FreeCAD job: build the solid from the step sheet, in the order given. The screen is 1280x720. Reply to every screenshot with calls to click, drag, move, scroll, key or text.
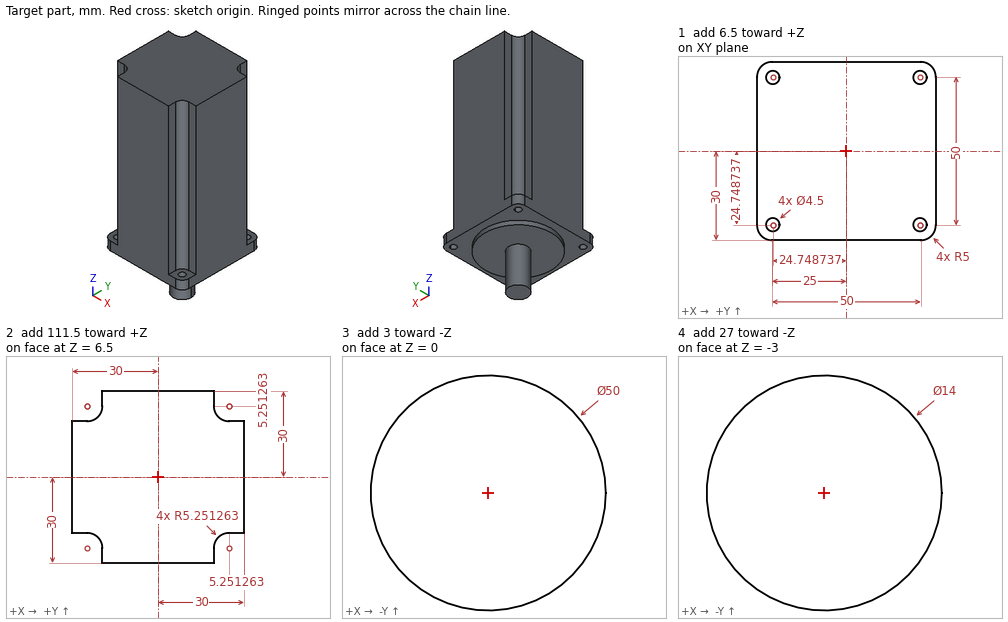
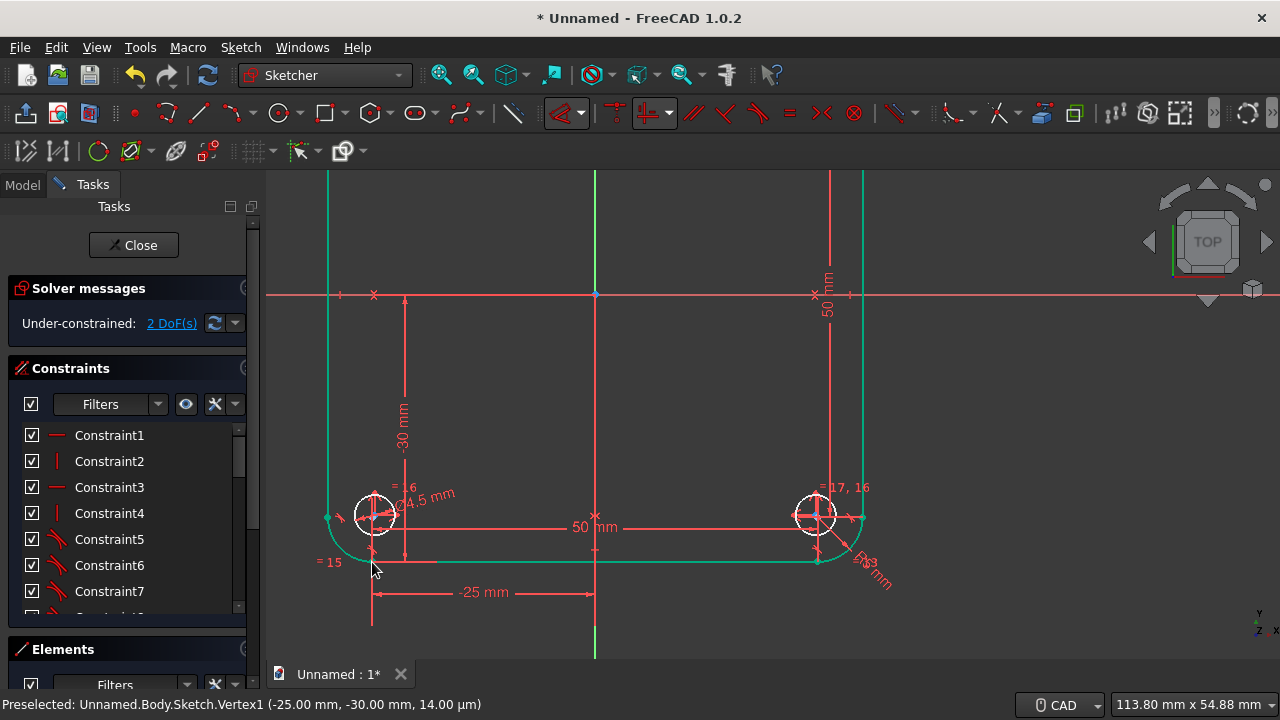
scroll(375, 515, up, 7)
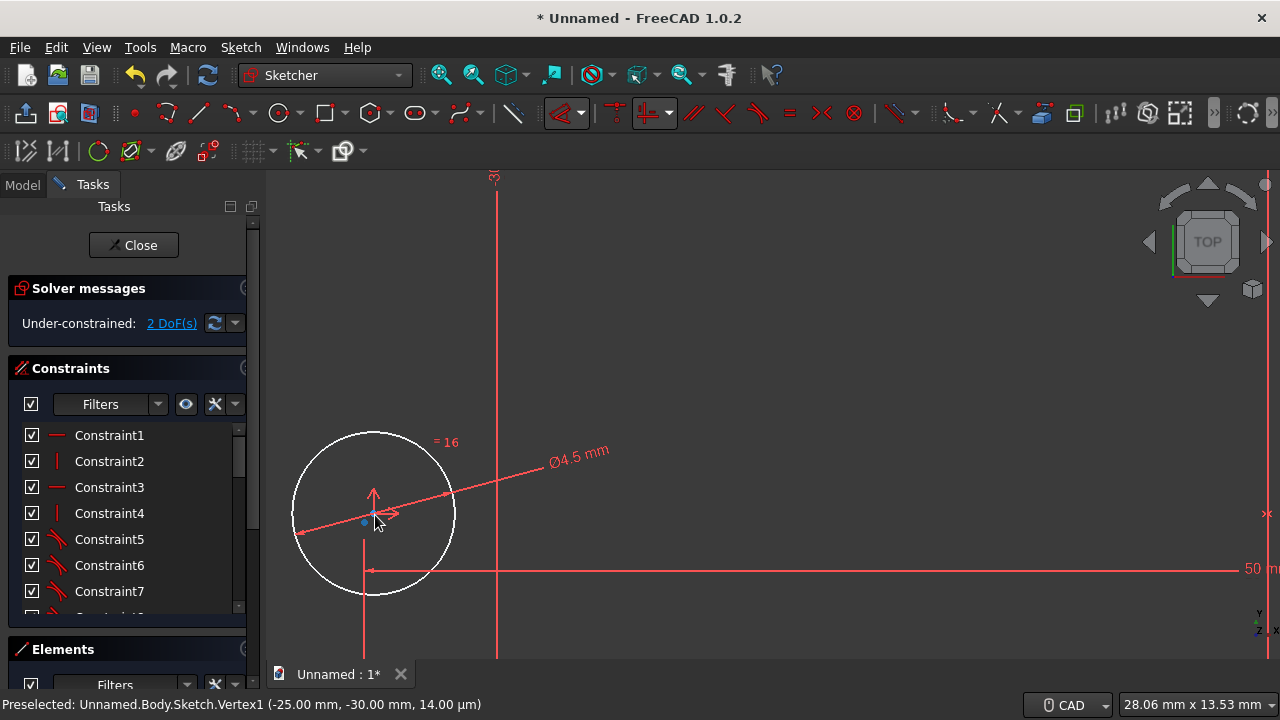
click(374, 514)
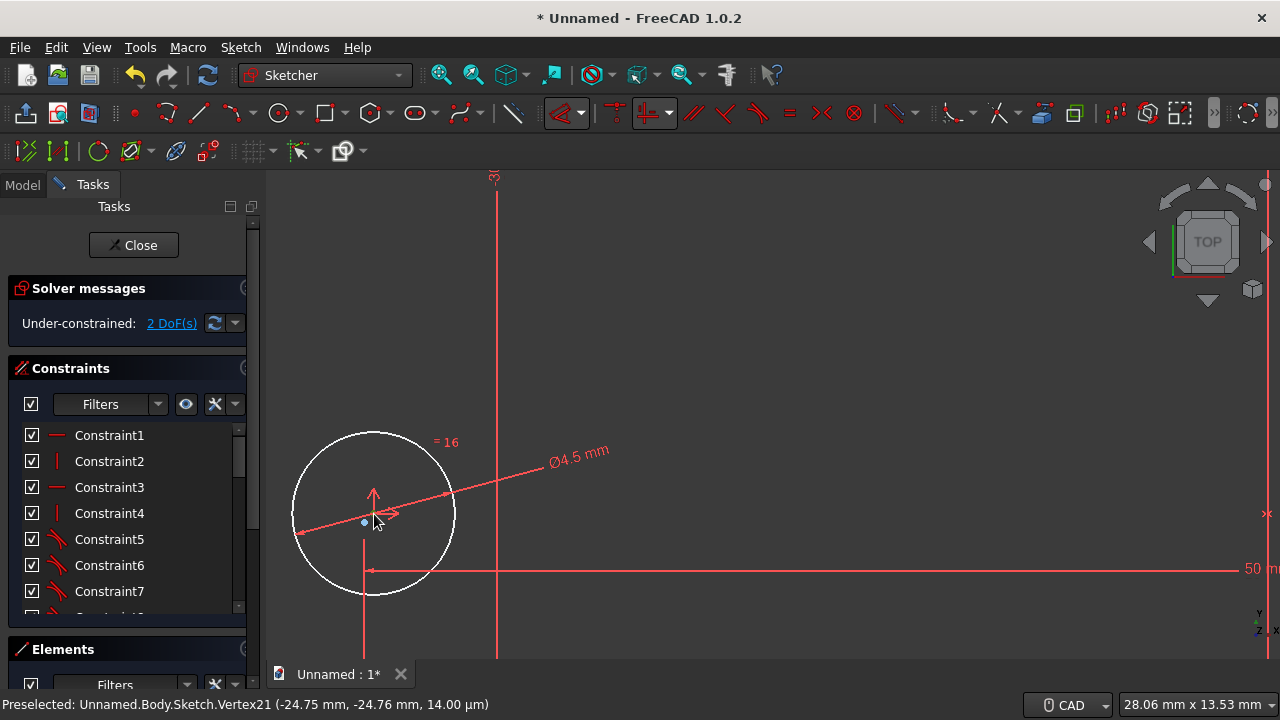
key(l)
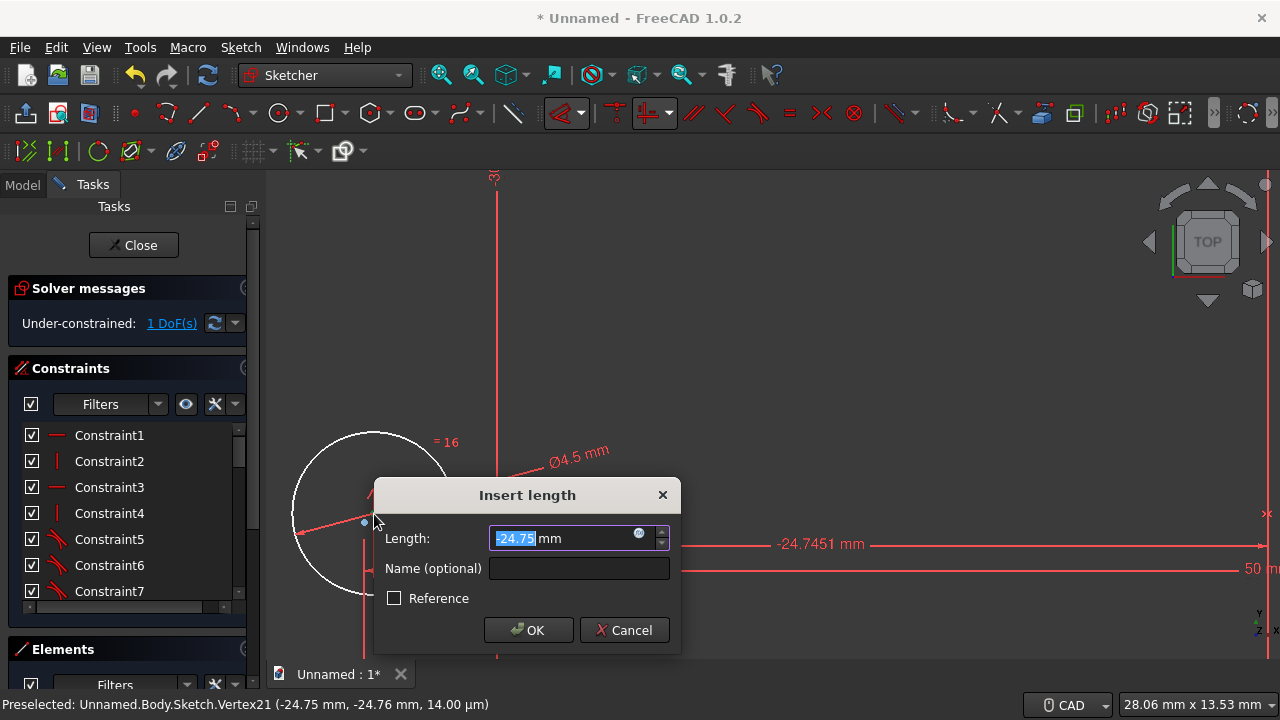
text(-24.748737)
key(Return)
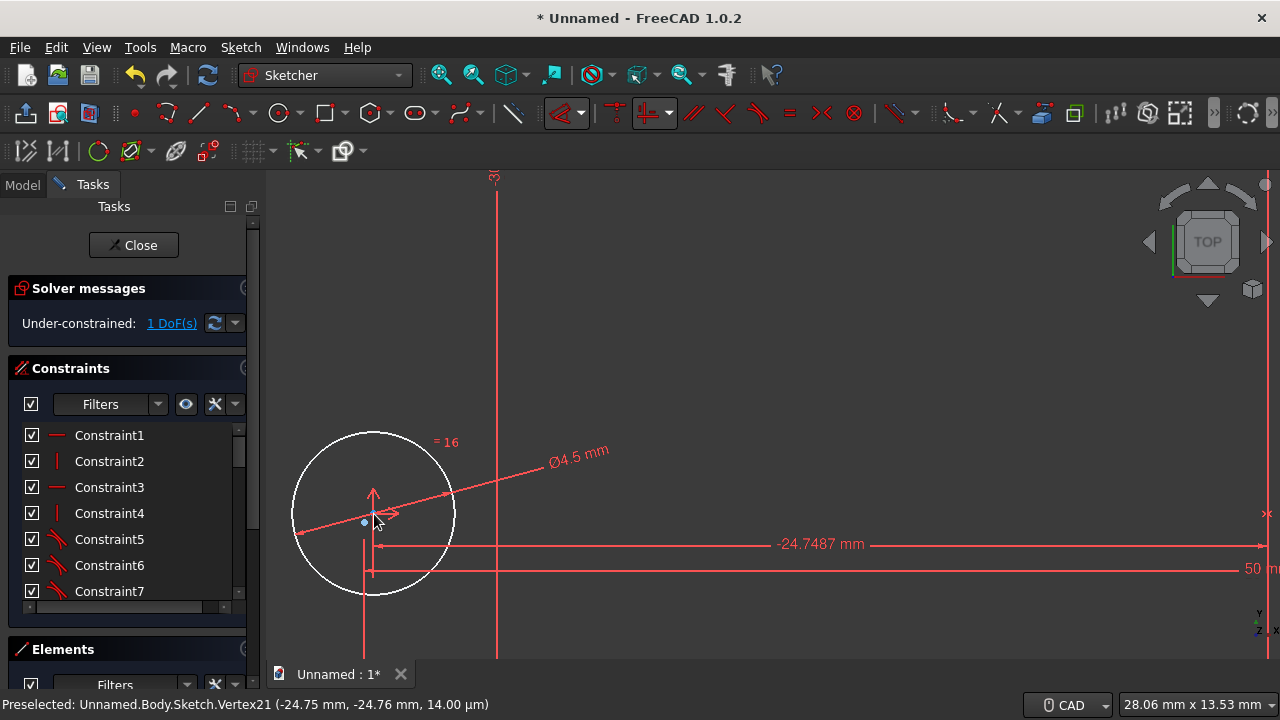
click(373, 514)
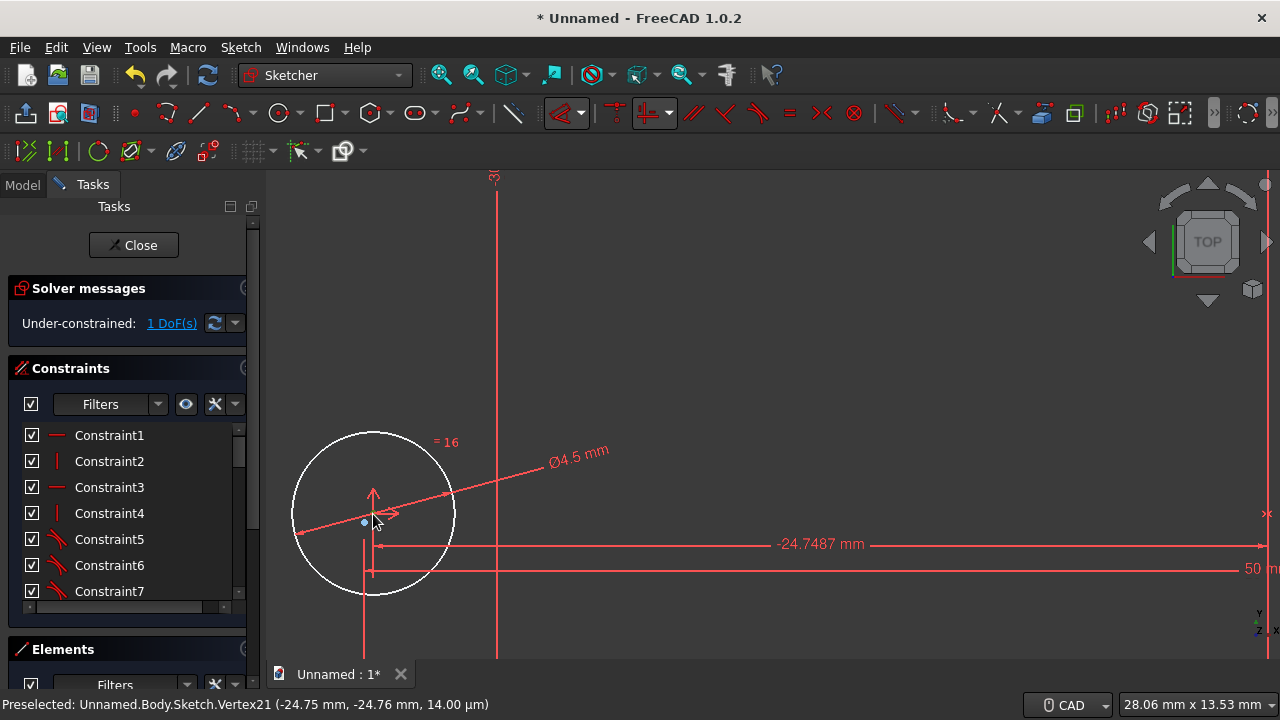
click(584, 114)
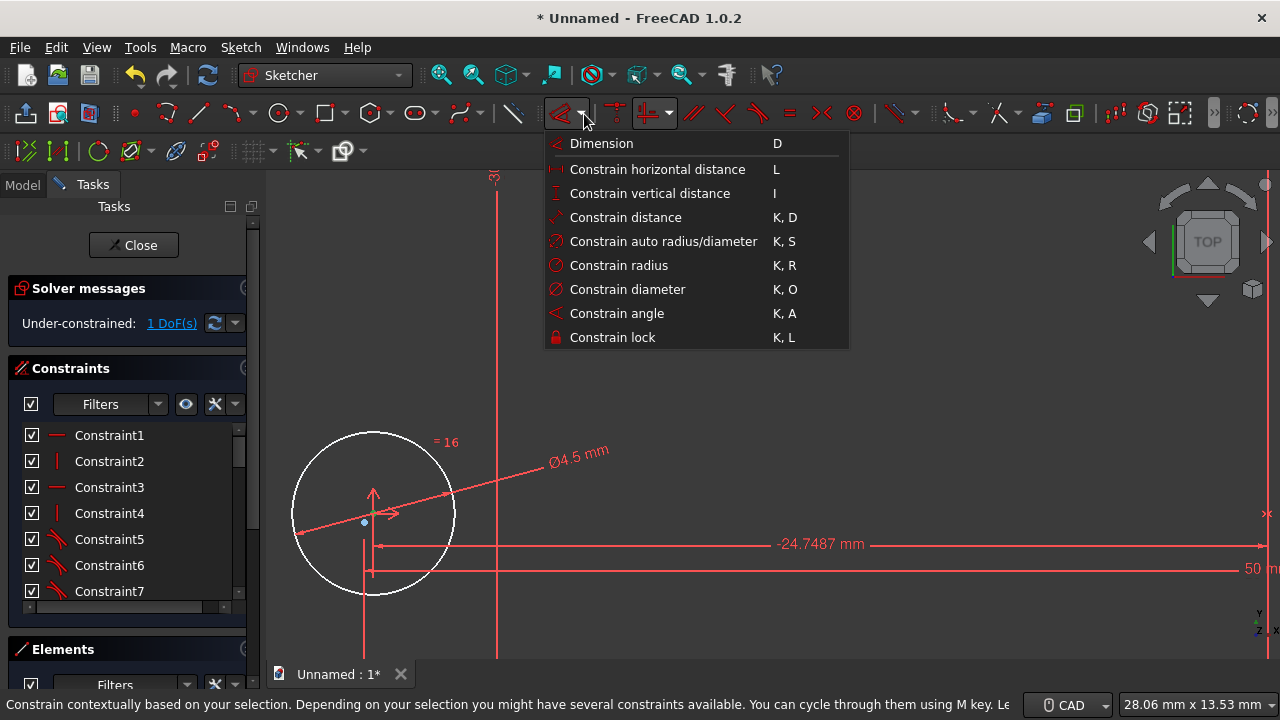
click(697, 193)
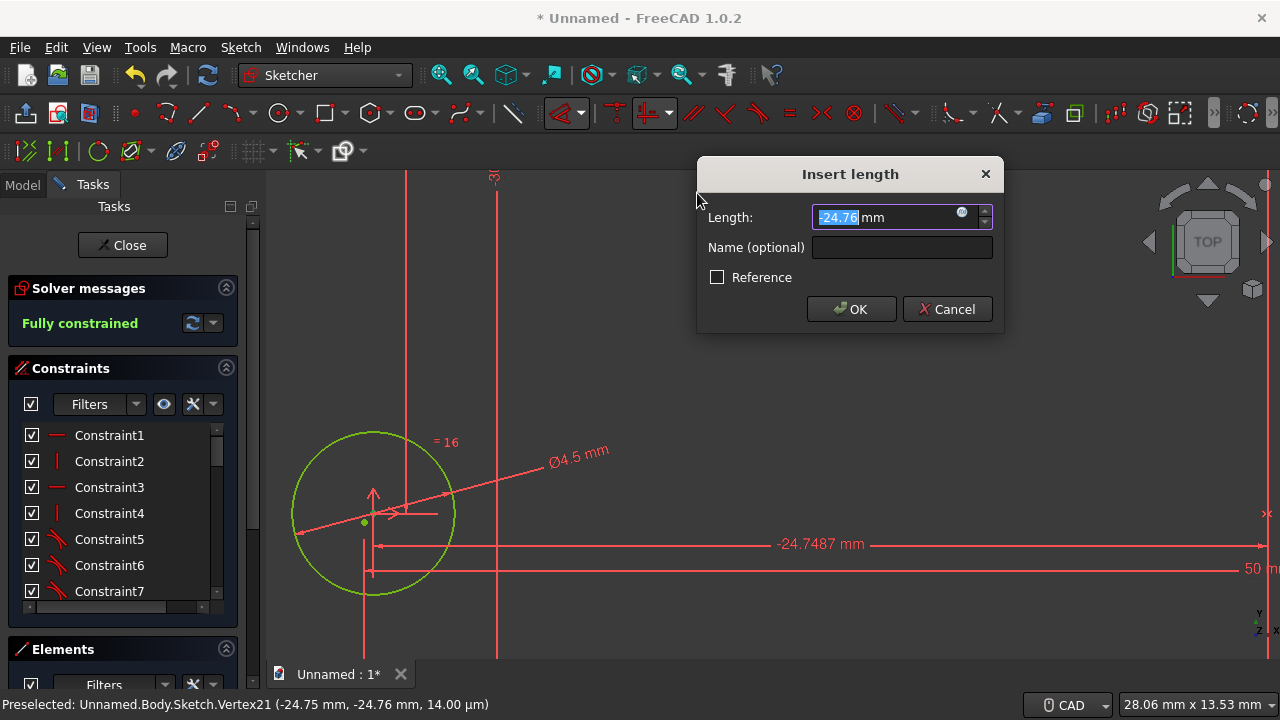
text(-24.748737)
key(Return)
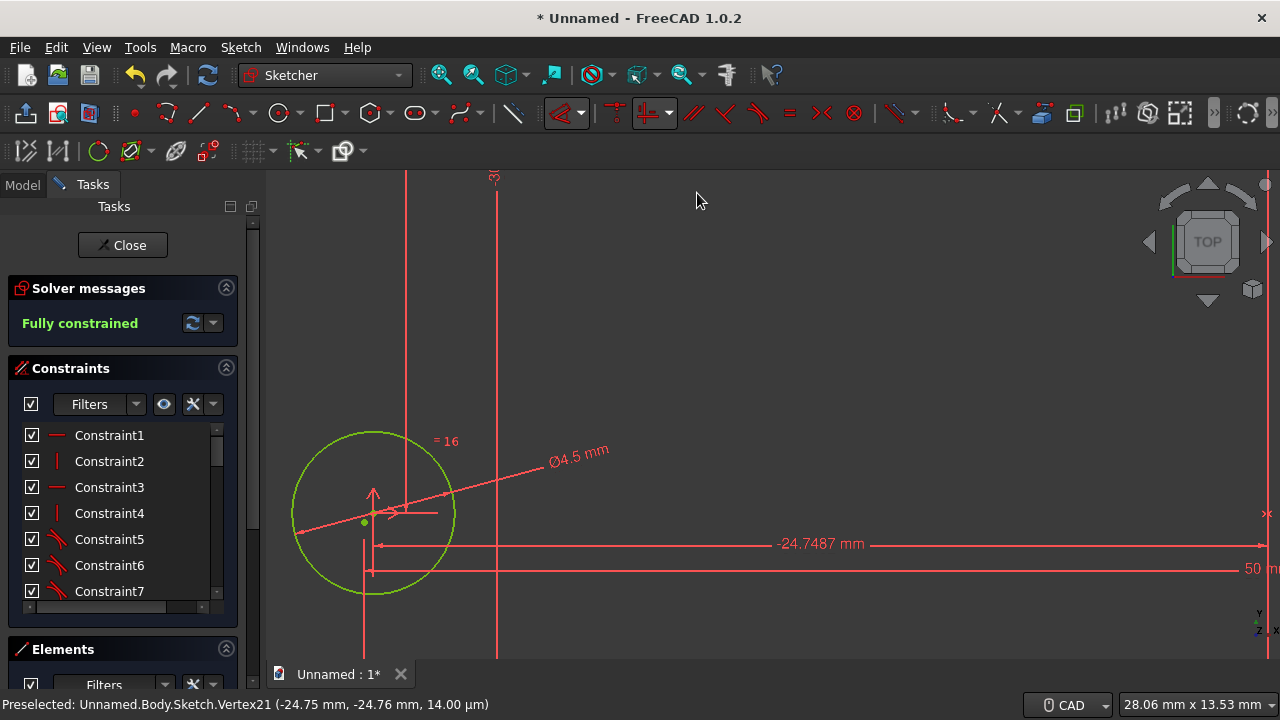
click(123, 245)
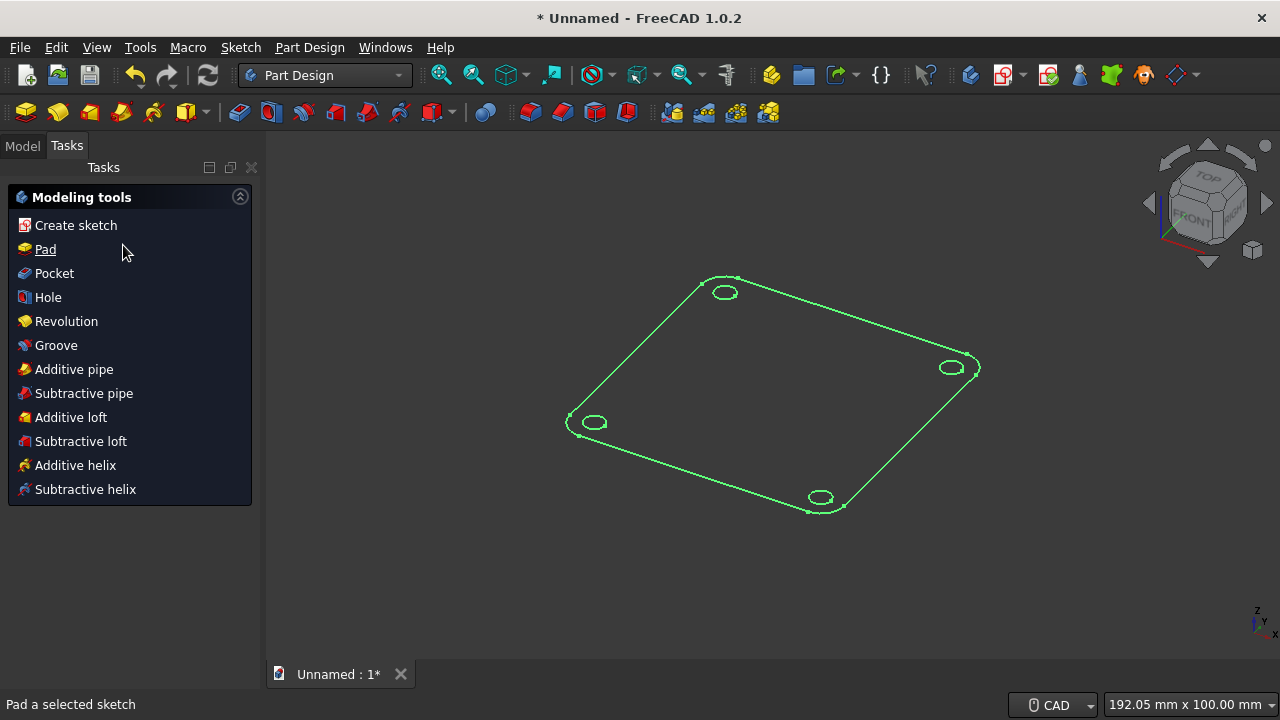
click(26, 112)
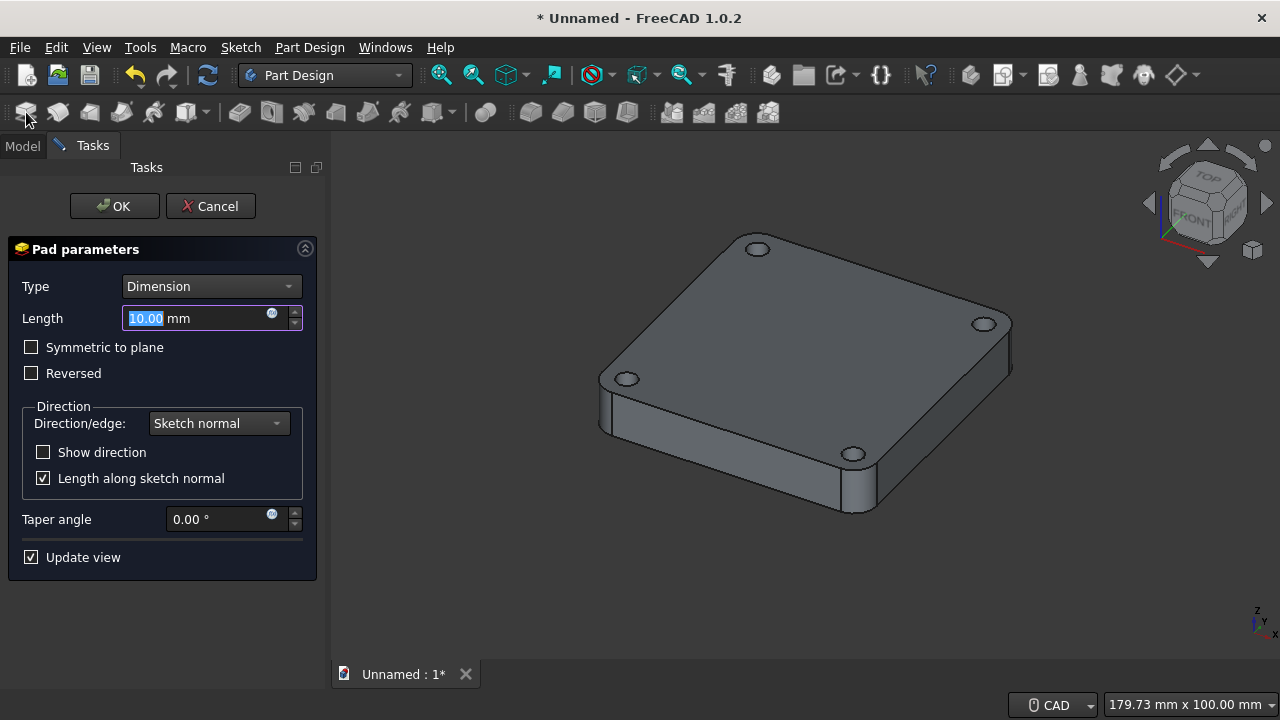
text(6.5)
key(Tab)